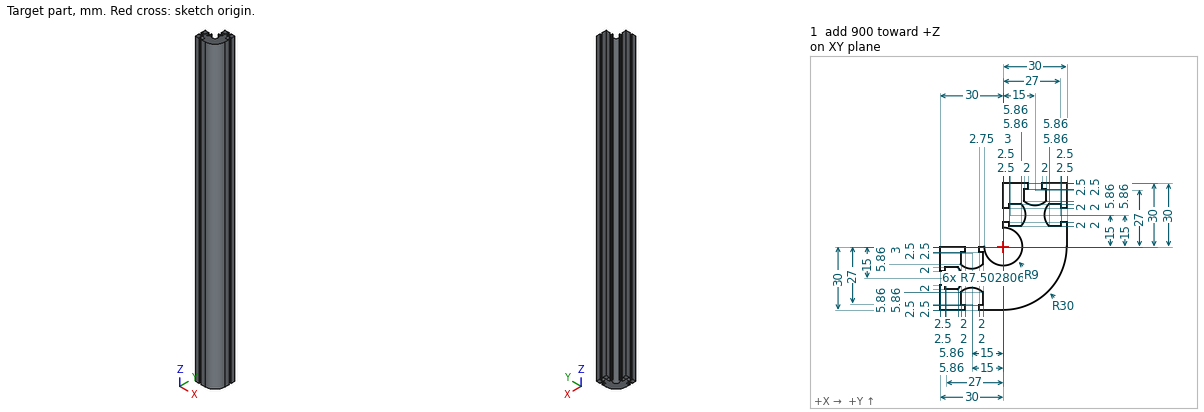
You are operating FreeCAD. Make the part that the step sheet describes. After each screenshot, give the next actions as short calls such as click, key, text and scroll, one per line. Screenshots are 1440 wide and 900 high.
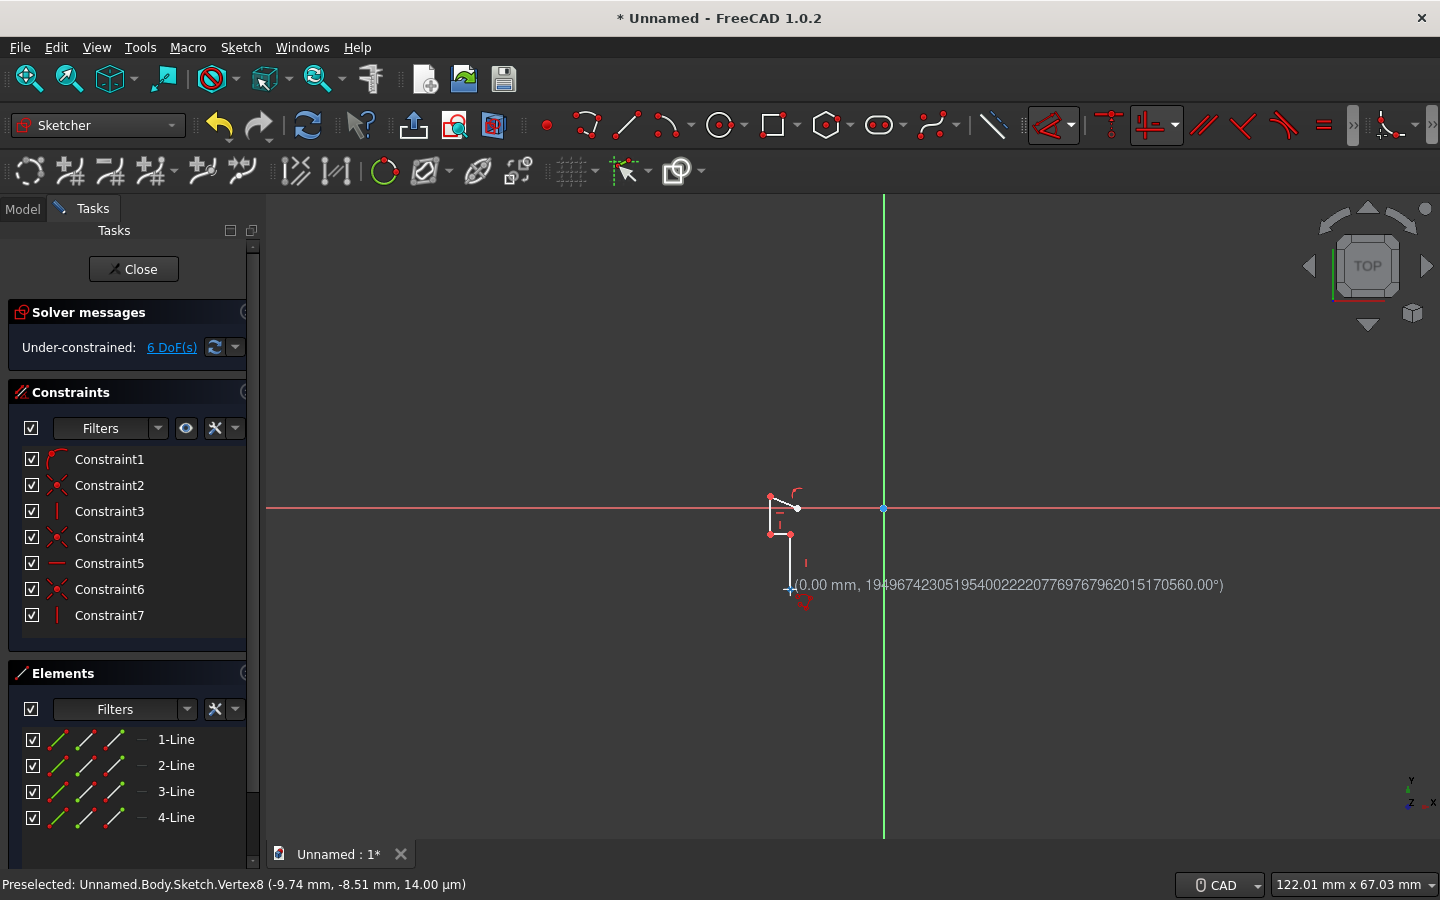
click(689, 589)
click(689, 532)
click(708, 532)
click(708, 508)
click(595, 499)
click(595, 621)
click(619, 621)
click(619, 602)
click(676, 602)
right_click(676, 602)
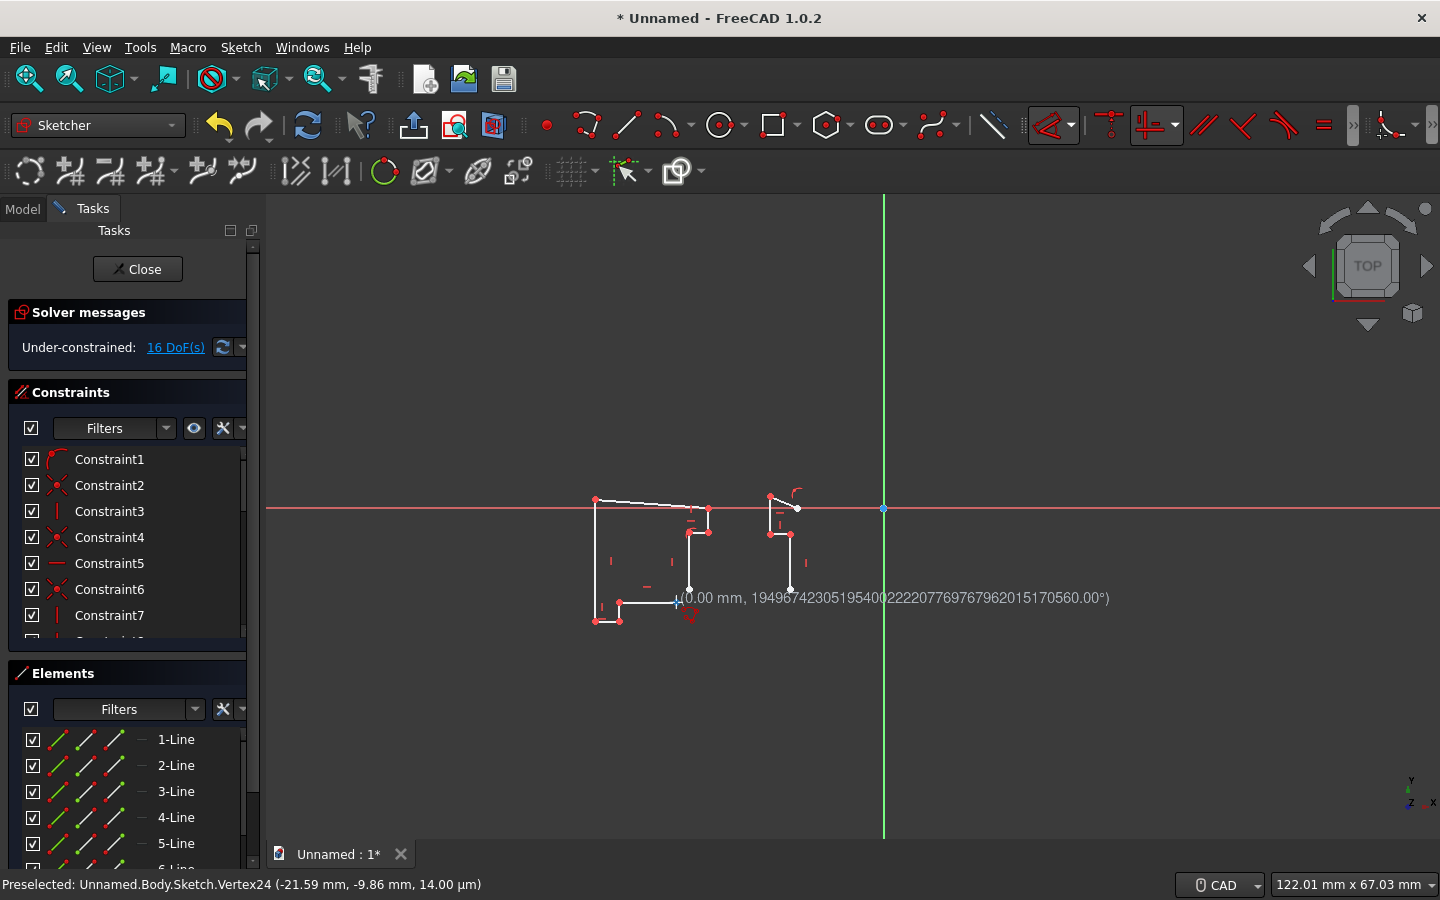
click(676, 703)
click(619, 703)
click(619, 684)
click(595, 684)
click(595, 797)
click(708, 797)
click(708, 773)
click(689, 773)
click(689, 716)
right_click(689, 716)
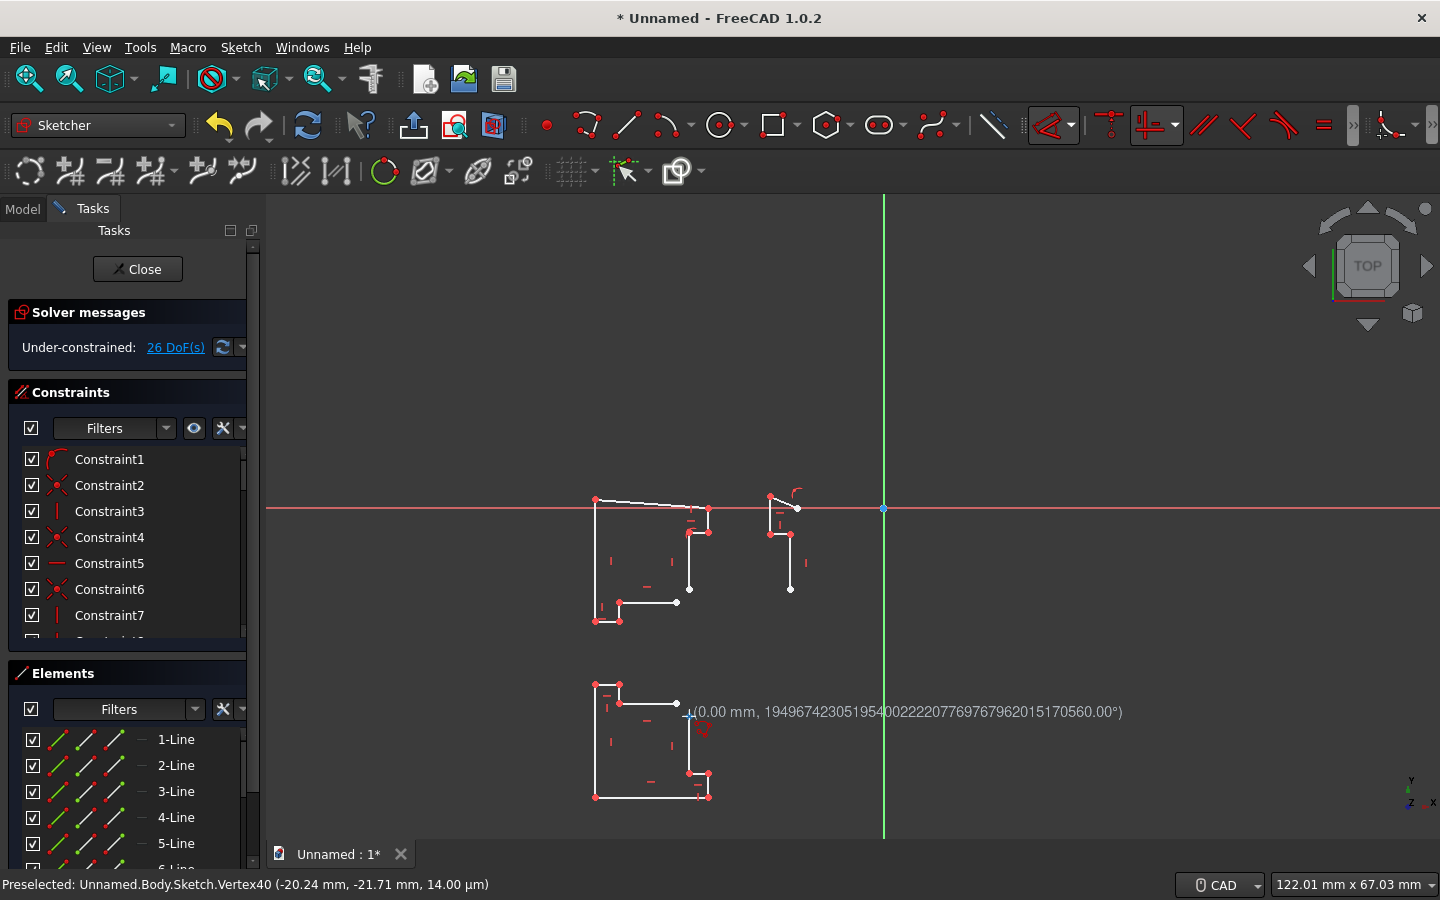
click(790, 716)
click(790, 773)
click(771, 773)
click(771, 797)
click(884, 797)
right_click(884, 797)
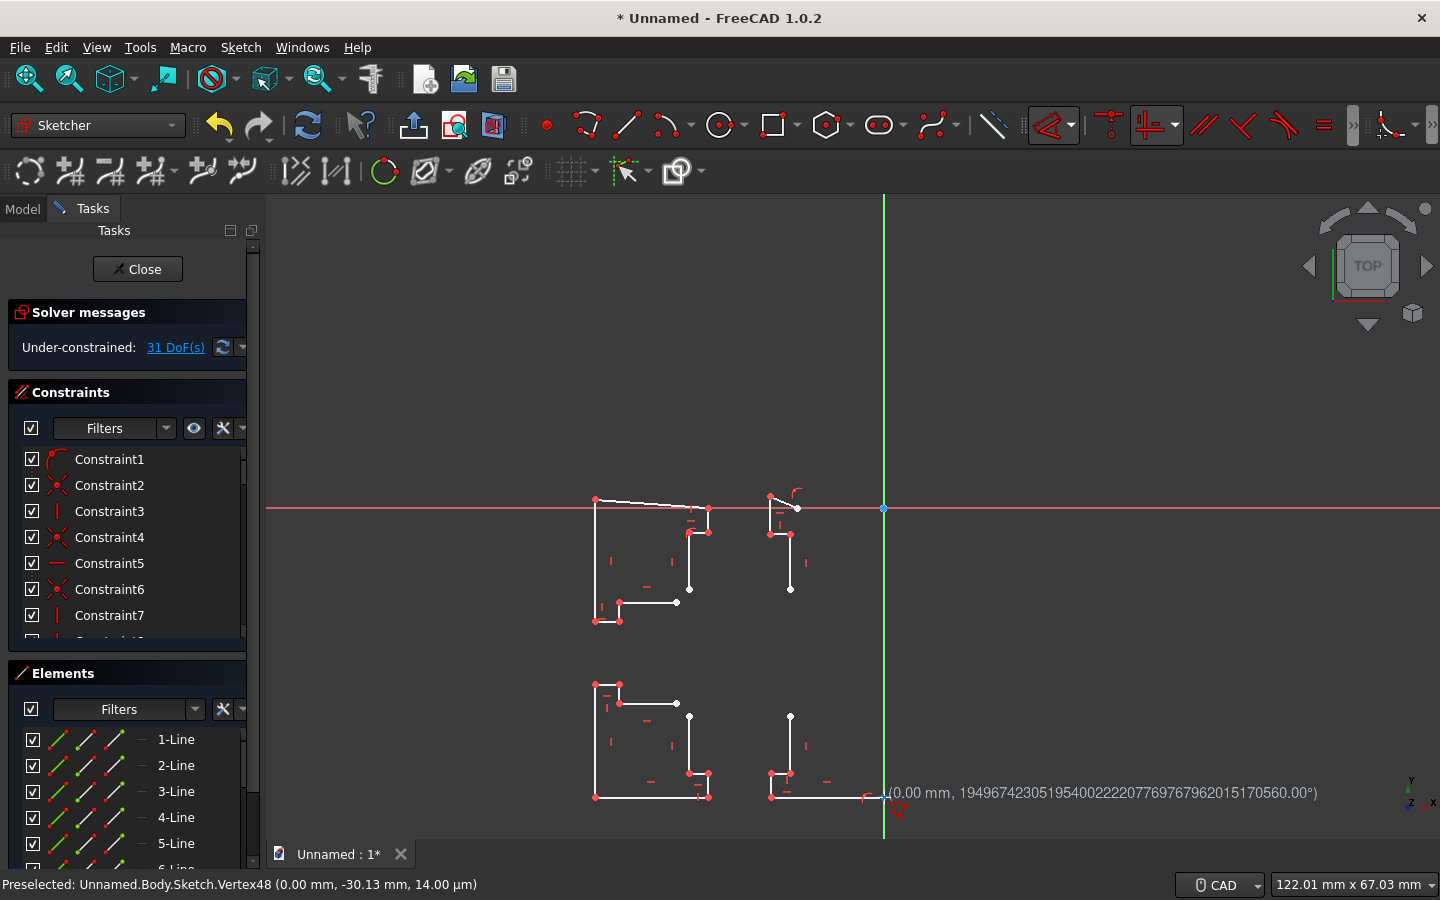
click(1172, 508)
click(1172, 395)
click(1148, 395)
click(1148, 414)
click(1092, 414)
right_click(1092, 414)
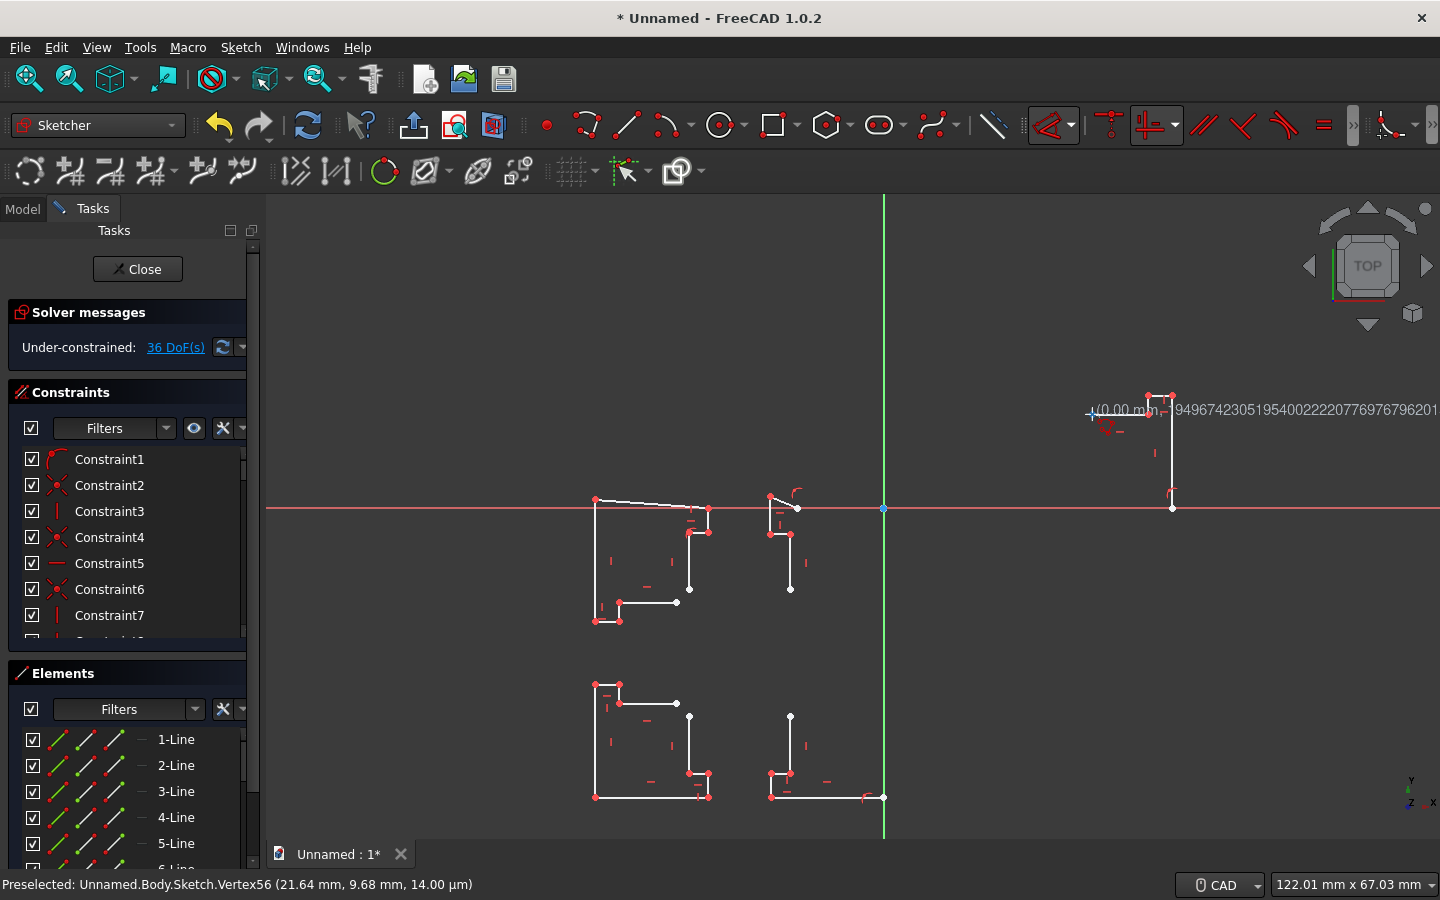
click(1092, 313)
click(1148, 313)
click(1148, 333)
click(1172, 333)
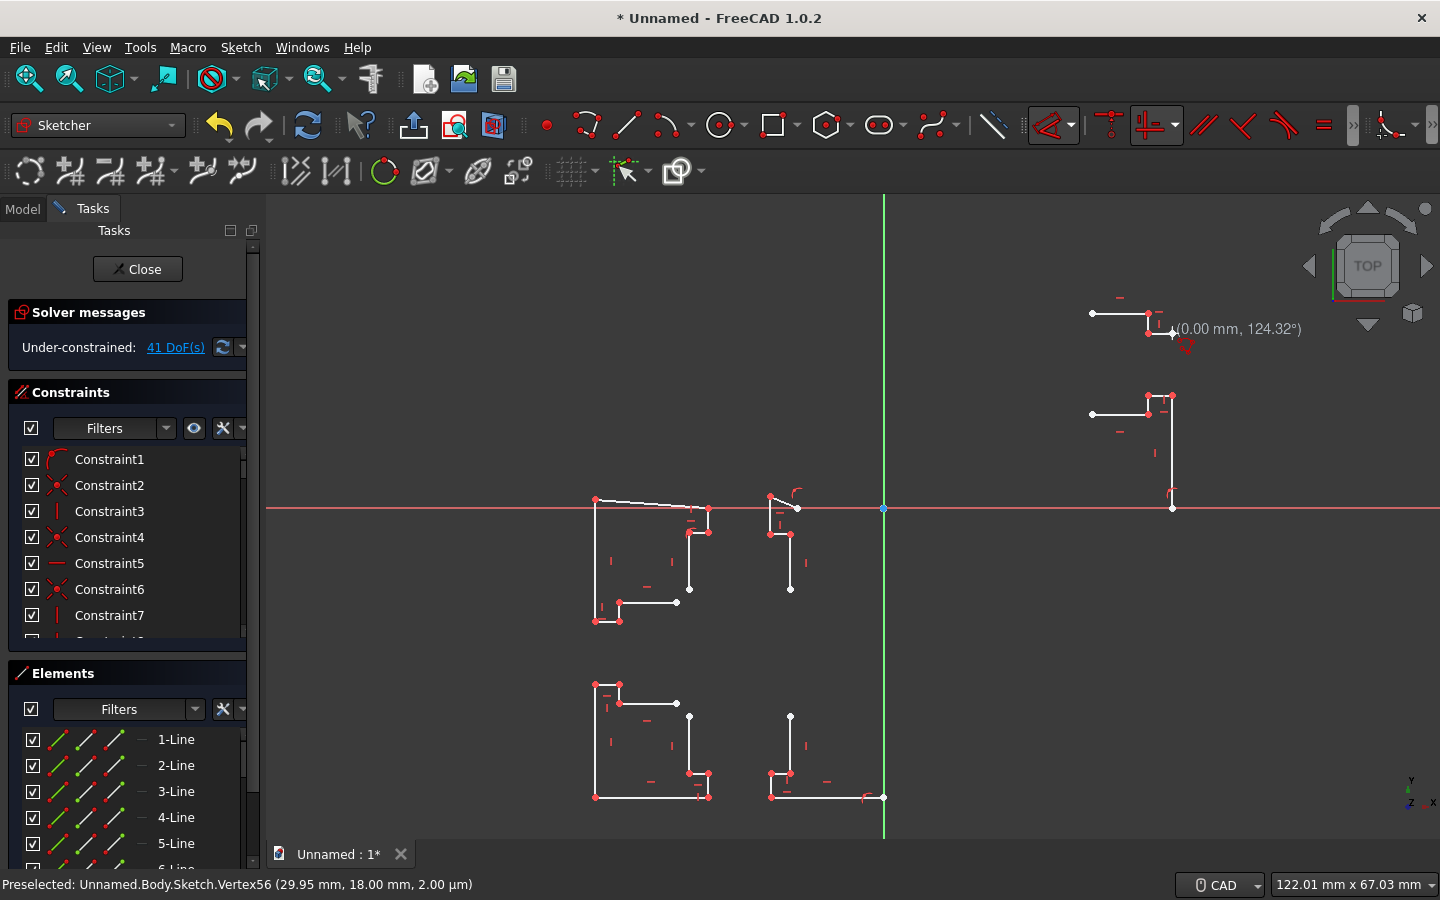
scroll(583, 534, down, 2)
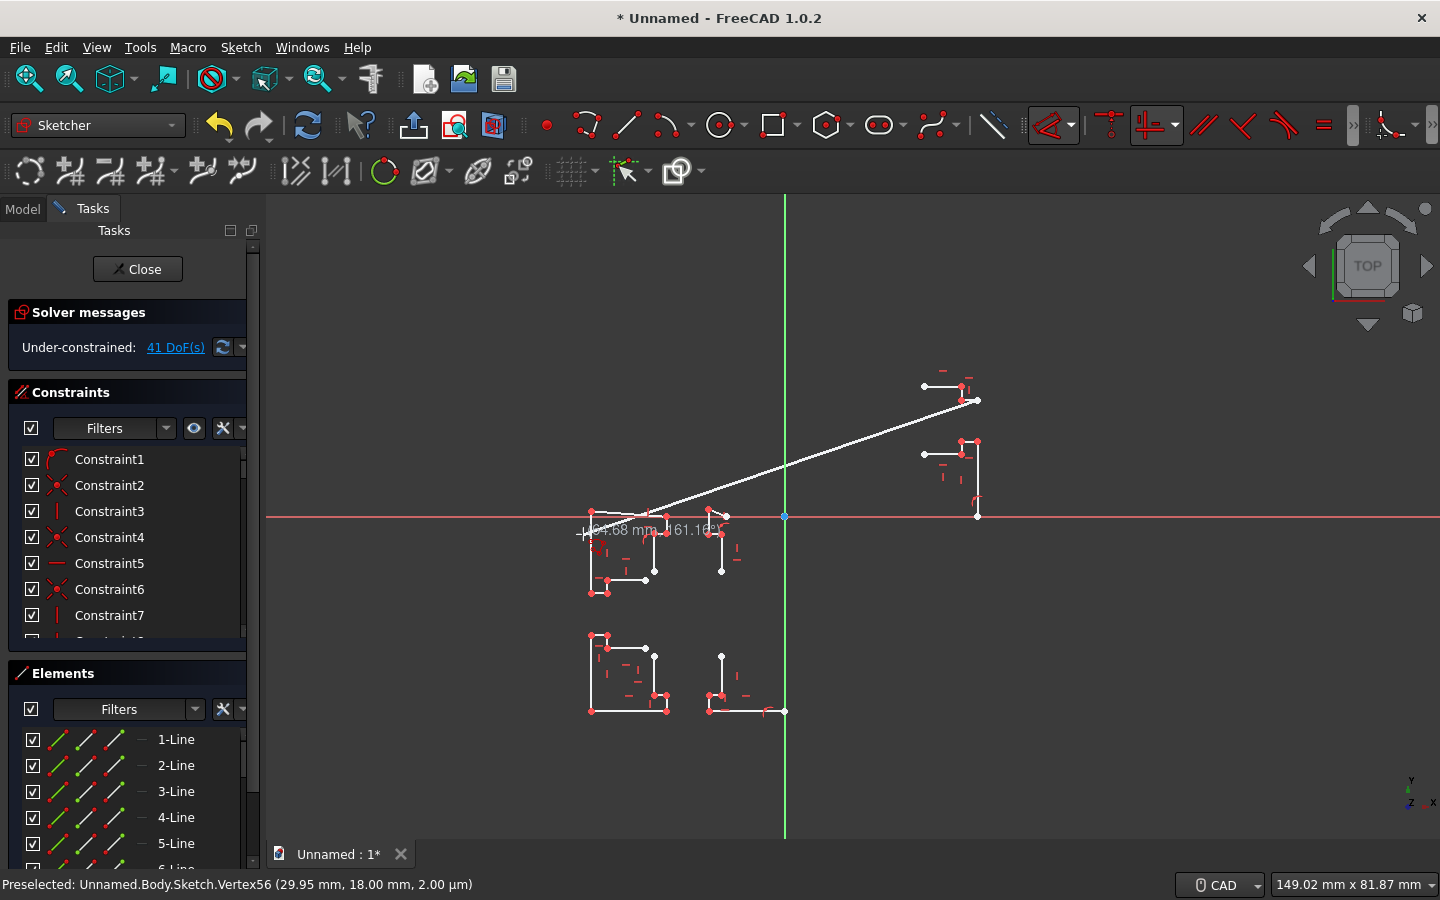
click(978, 323)
click(902, 323)
click(902, 339)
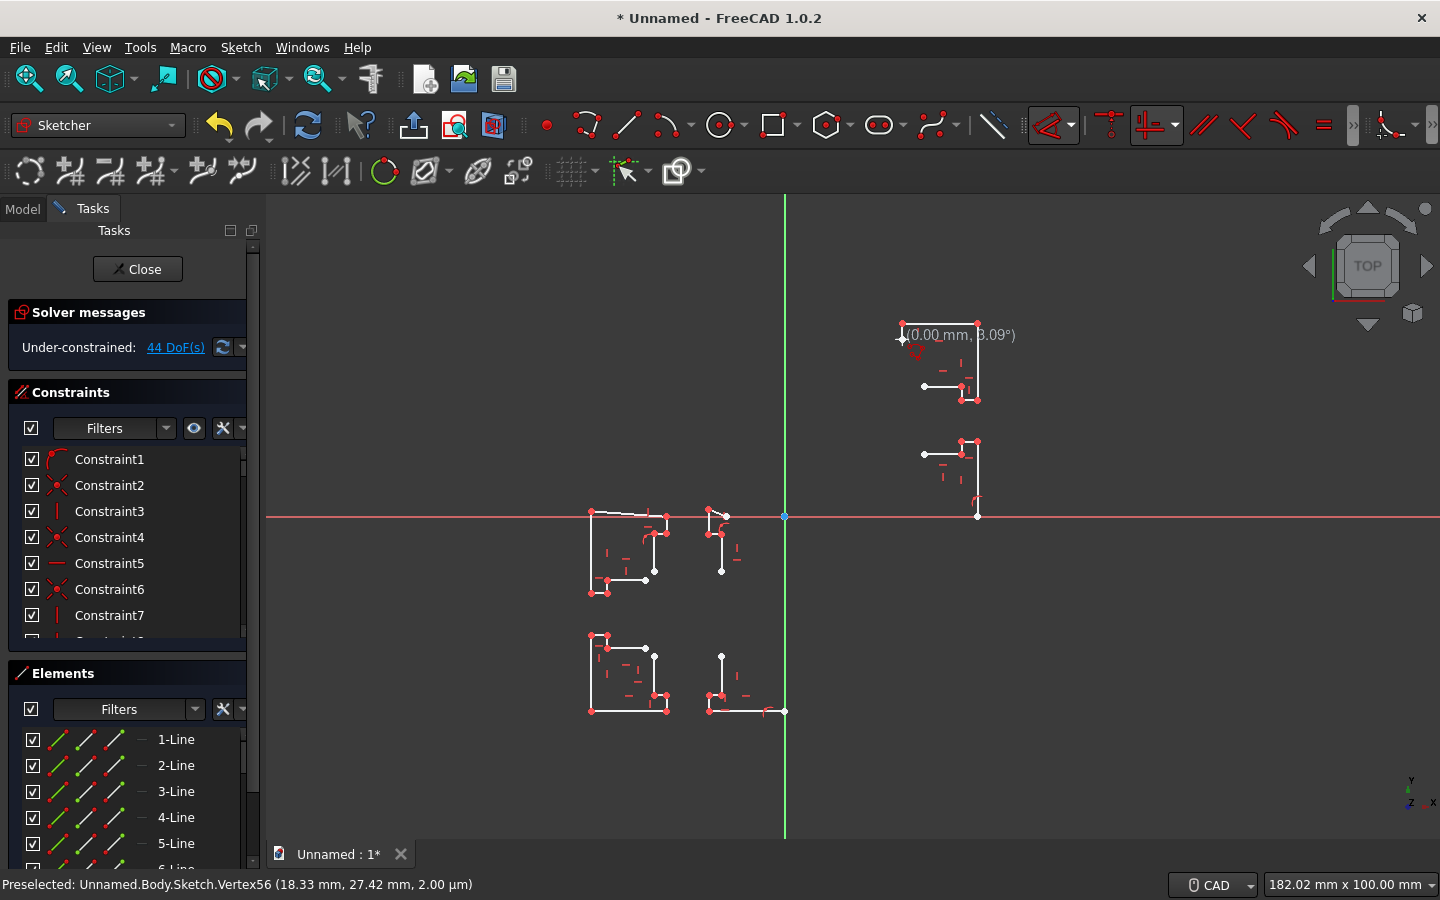
scroll(915, 339, up, 2)